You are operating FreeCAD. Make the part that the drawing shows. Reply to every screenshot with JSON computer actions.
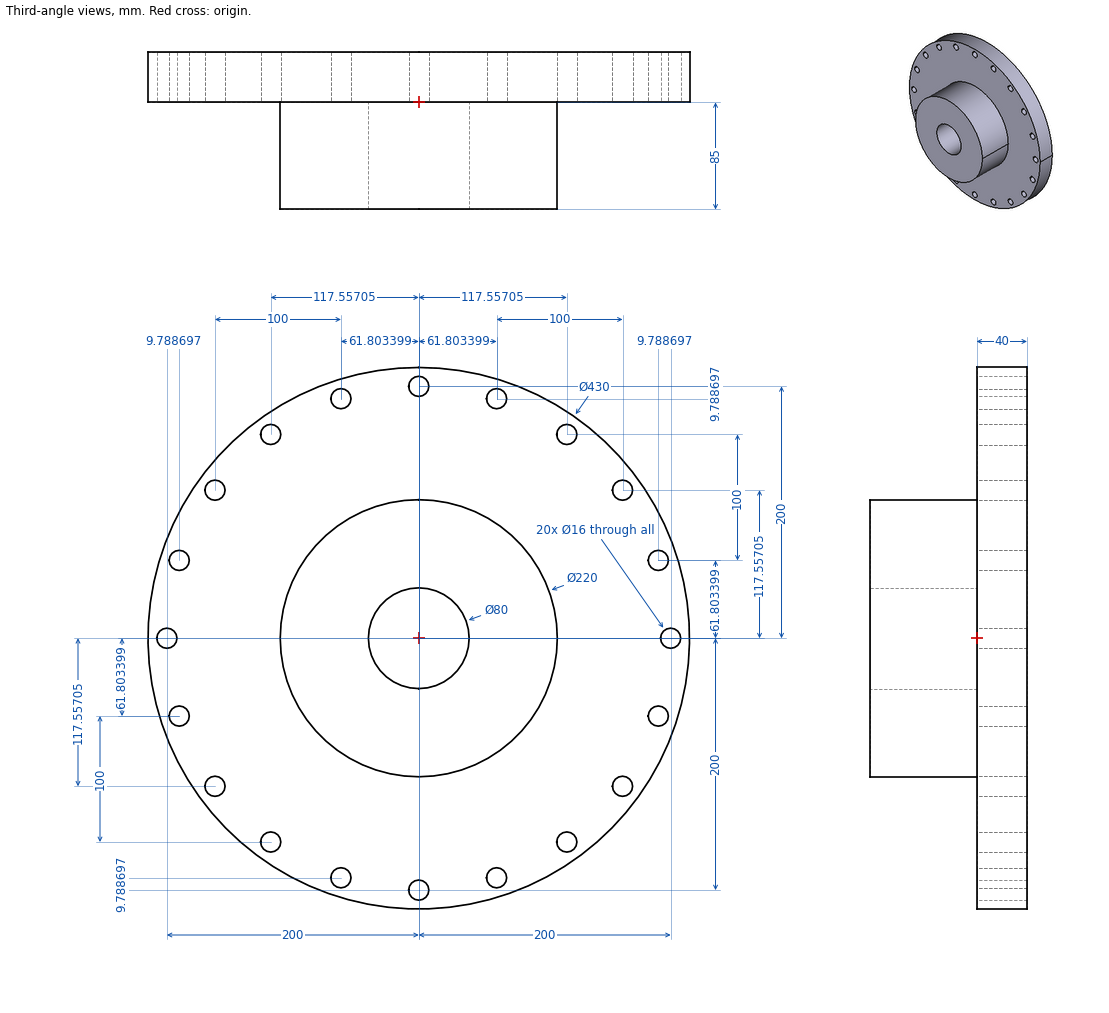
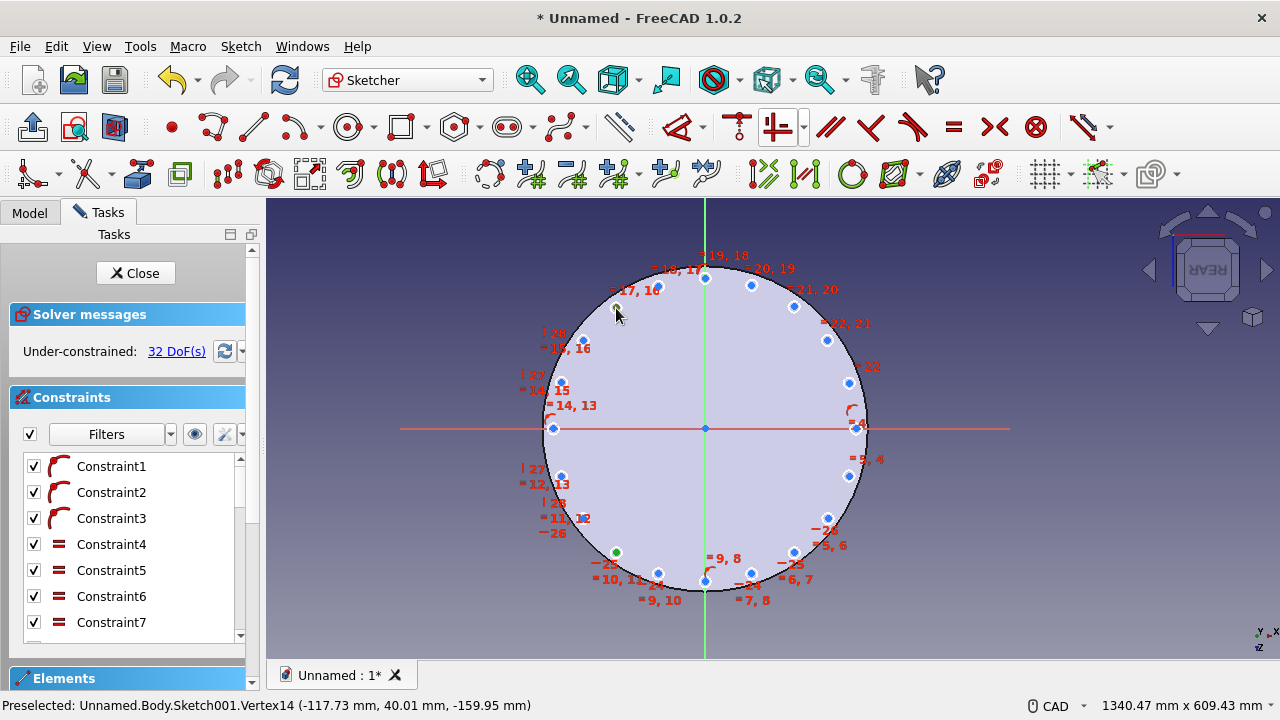
{"action": "key", "text": "v"}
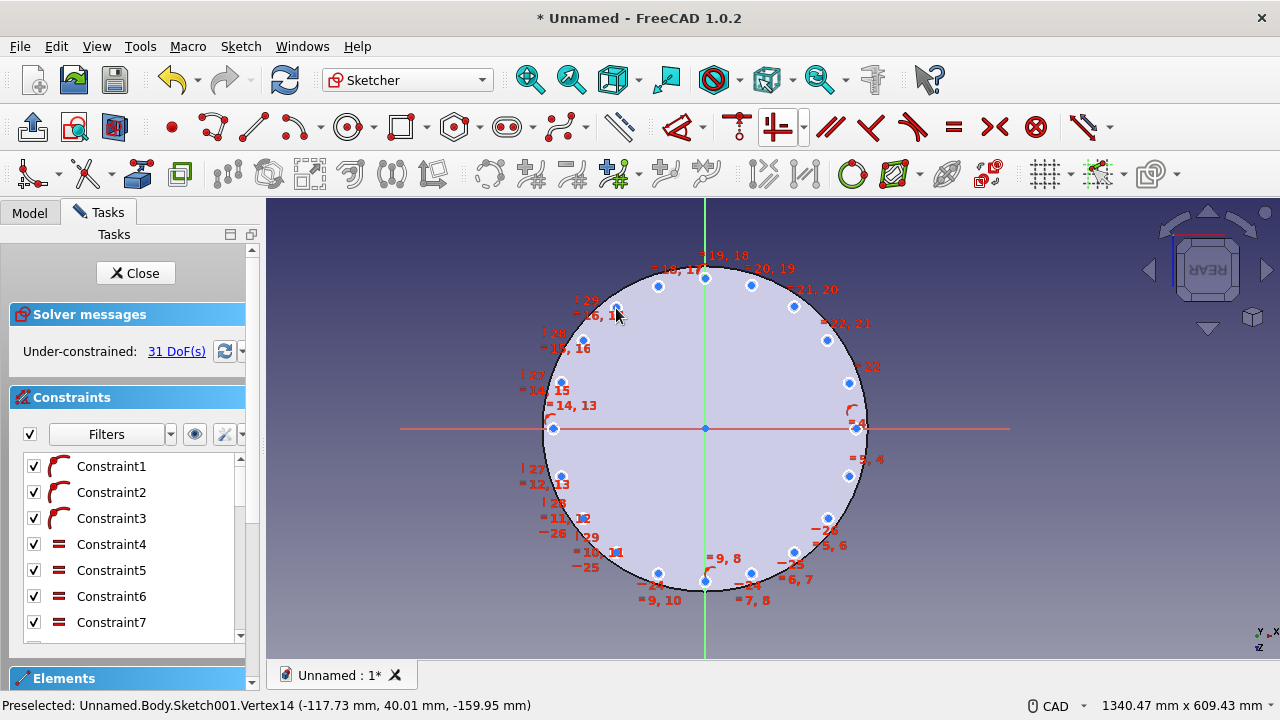
{"action": "left_click", "coordinate": [659, 286]}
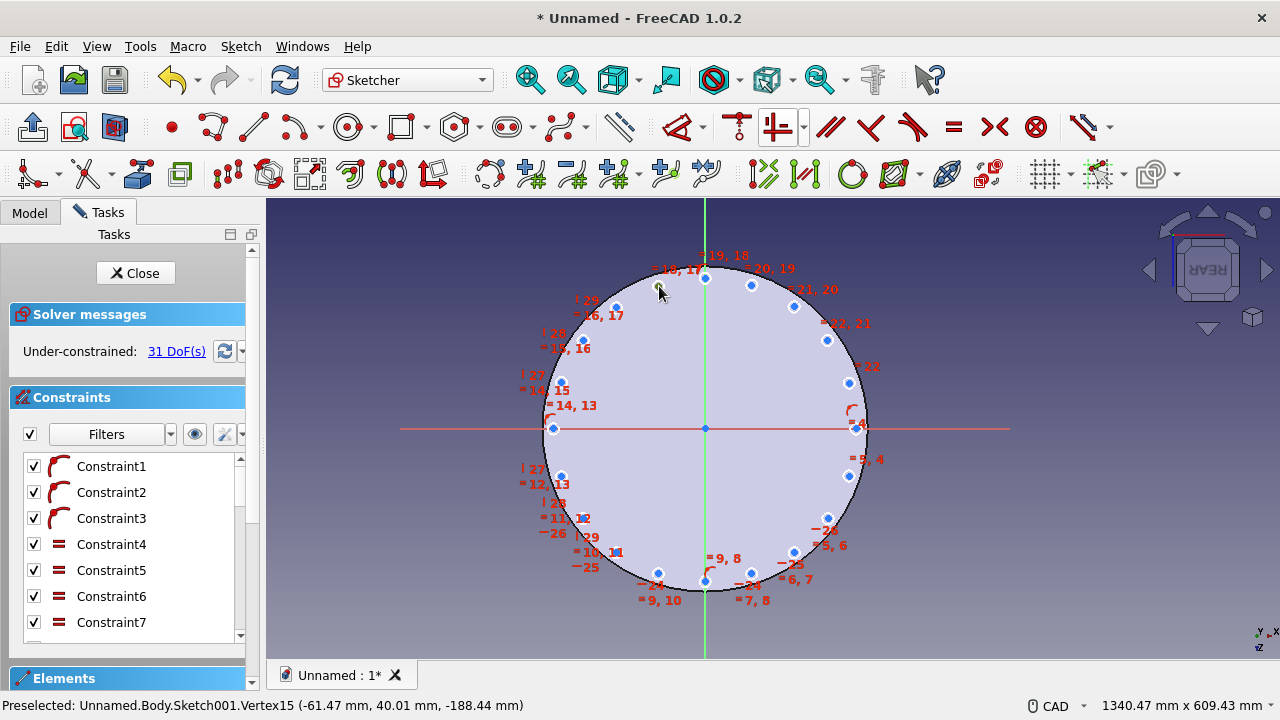
{"action": "left_click", "coordinate": [752, 285]}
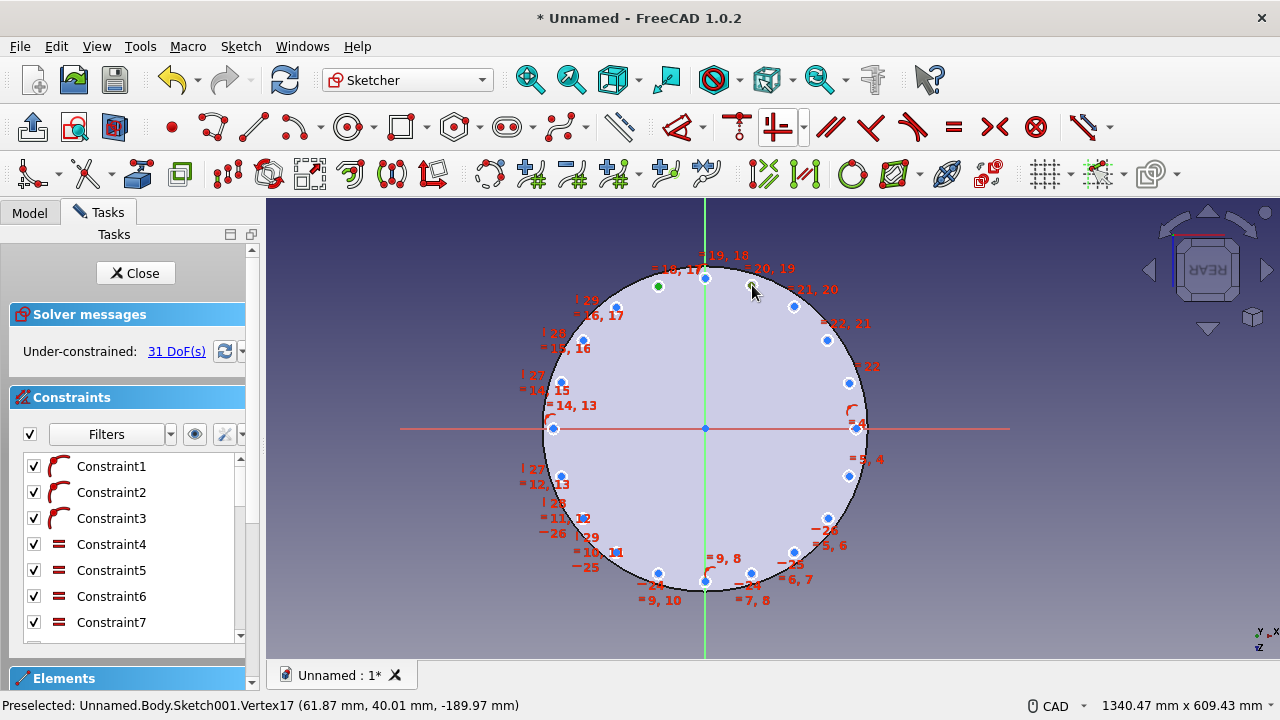
{"action": "key", "text": "h"}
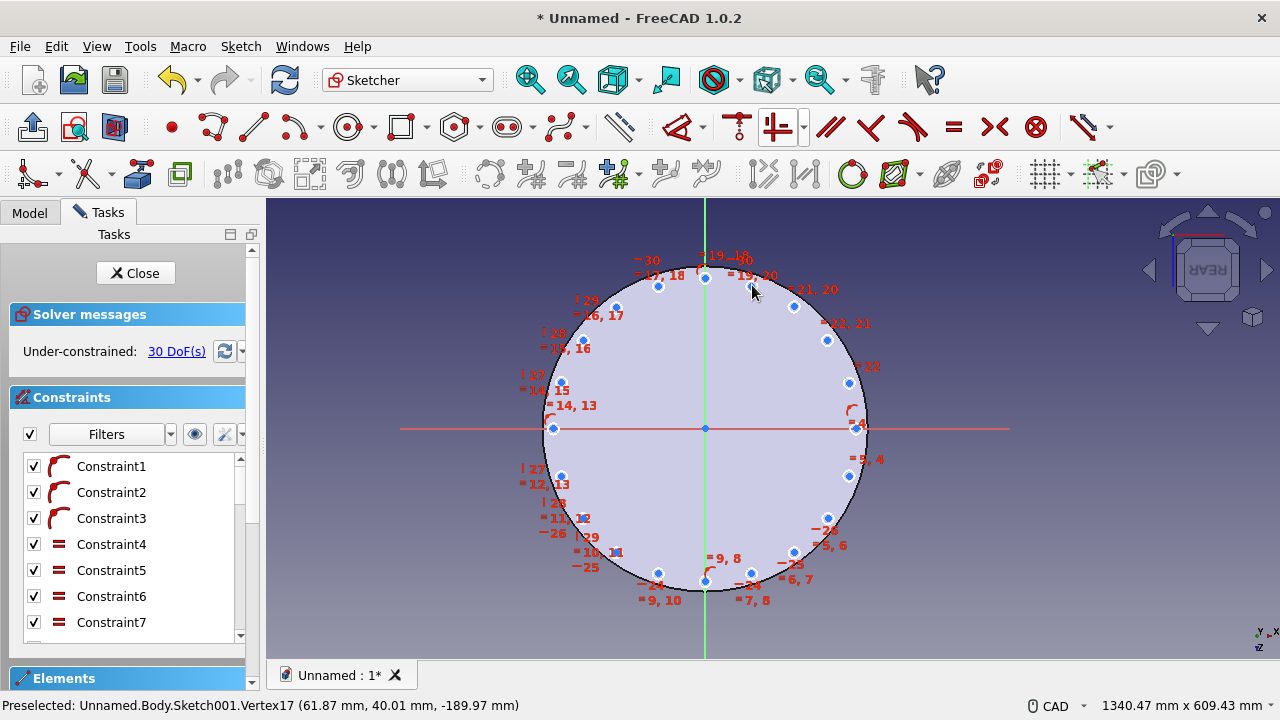
{"action": "scroll", "coordinate": [616, 308], "scroll_direction": "up", "scroll_amount": 4}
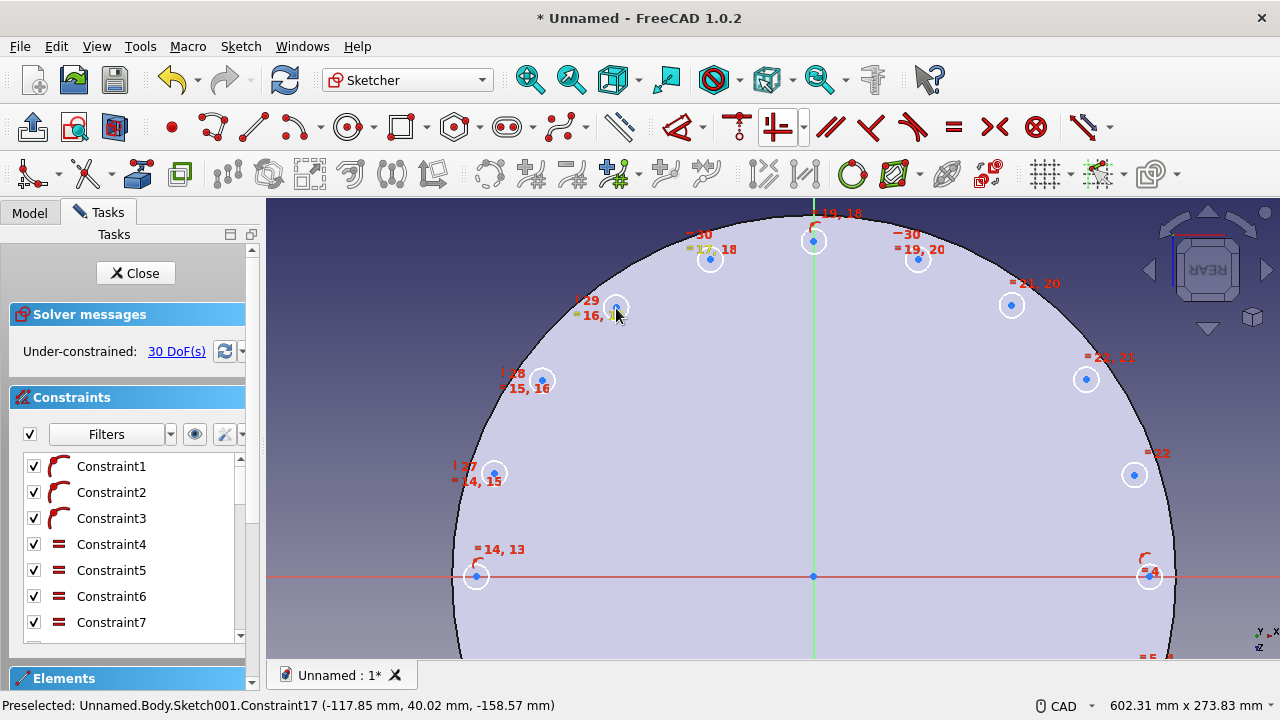
{"action": "scroll", "coordinate": [616, 308], "scroll_direction": "up", "scroll_amount": 4}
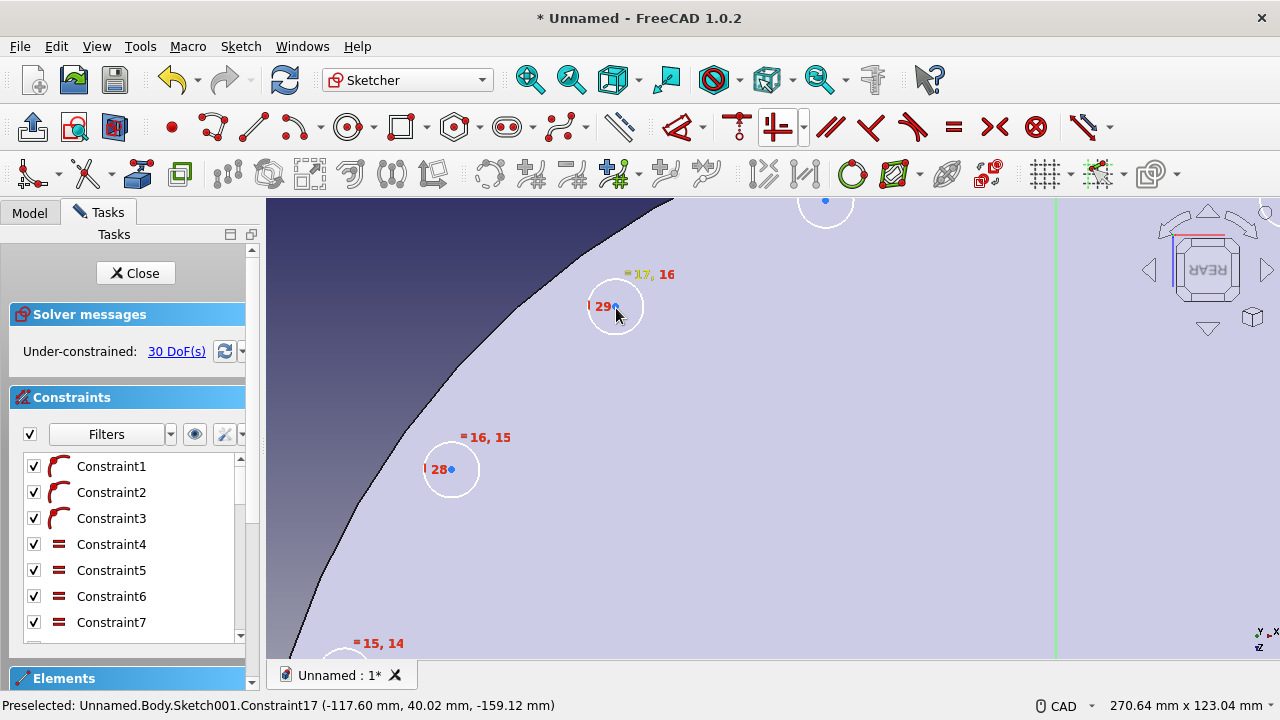
{"action": "left_click", "coordinate": [616, 307]}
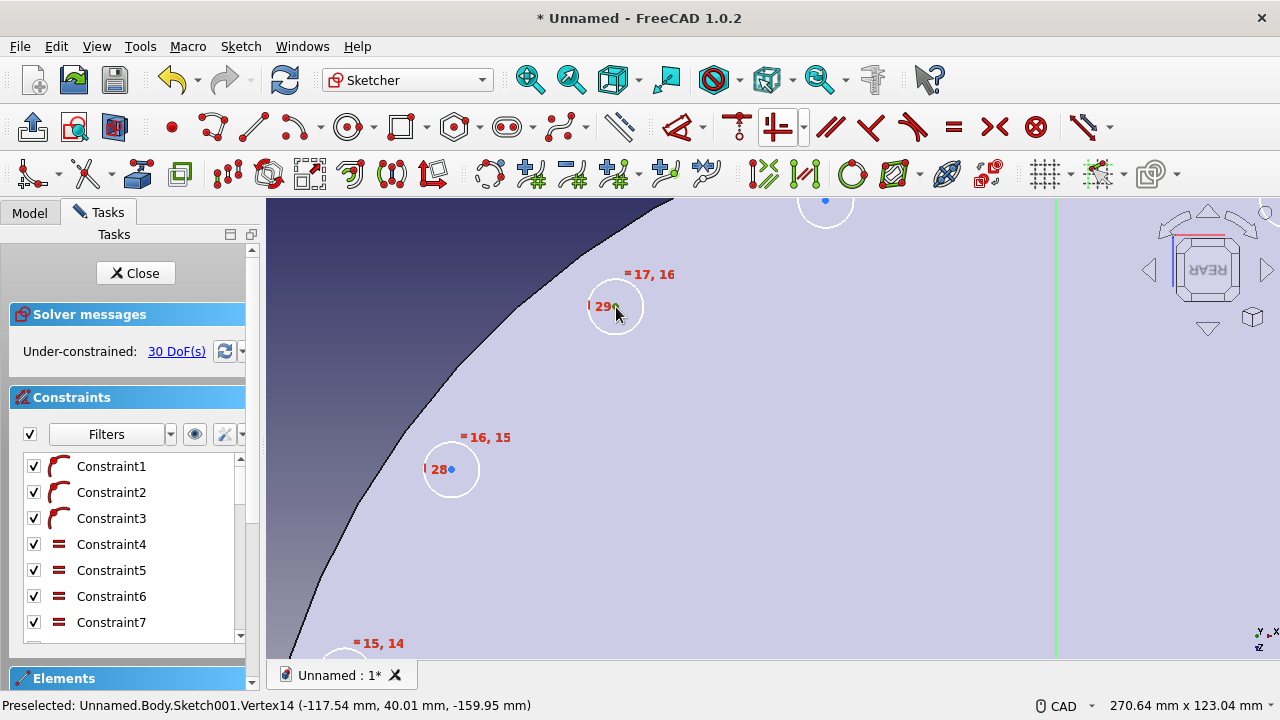
{"action": "scroll", "coordinate": [616, 308], "scroll_direction": "down", "scroll_amount": 8}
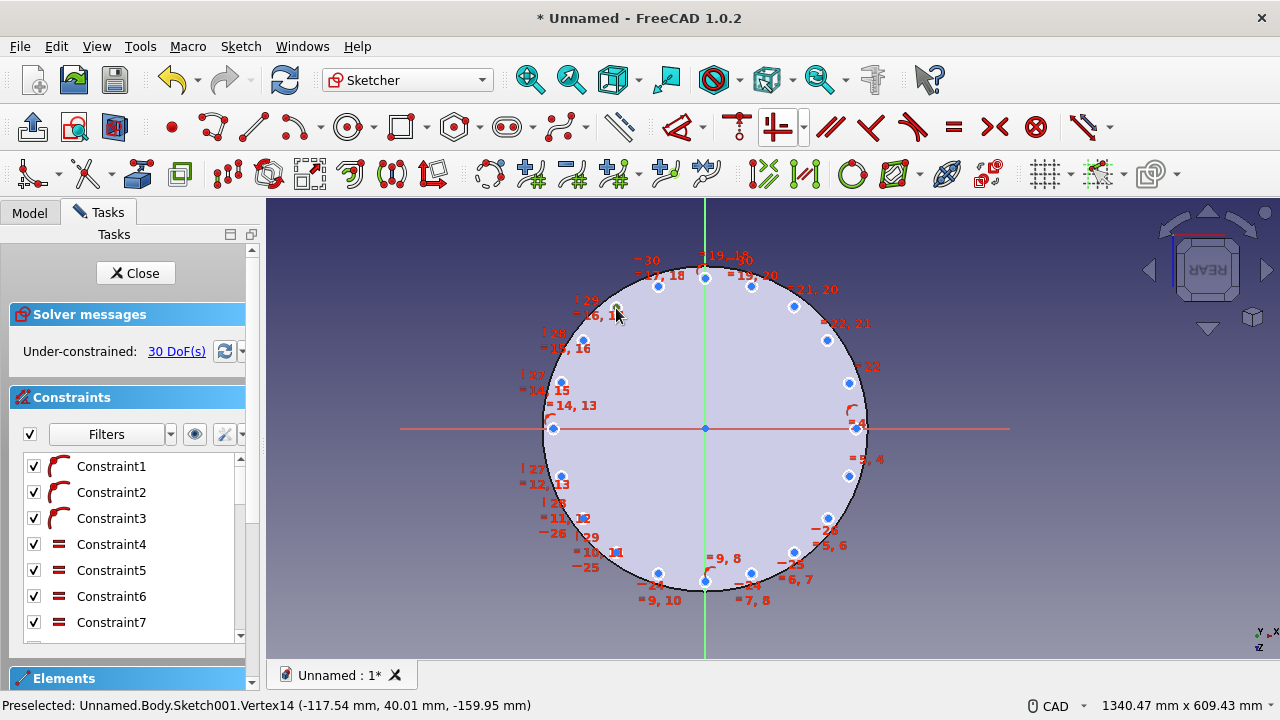
{"action": "left_click", "coordinate": [794, 307]}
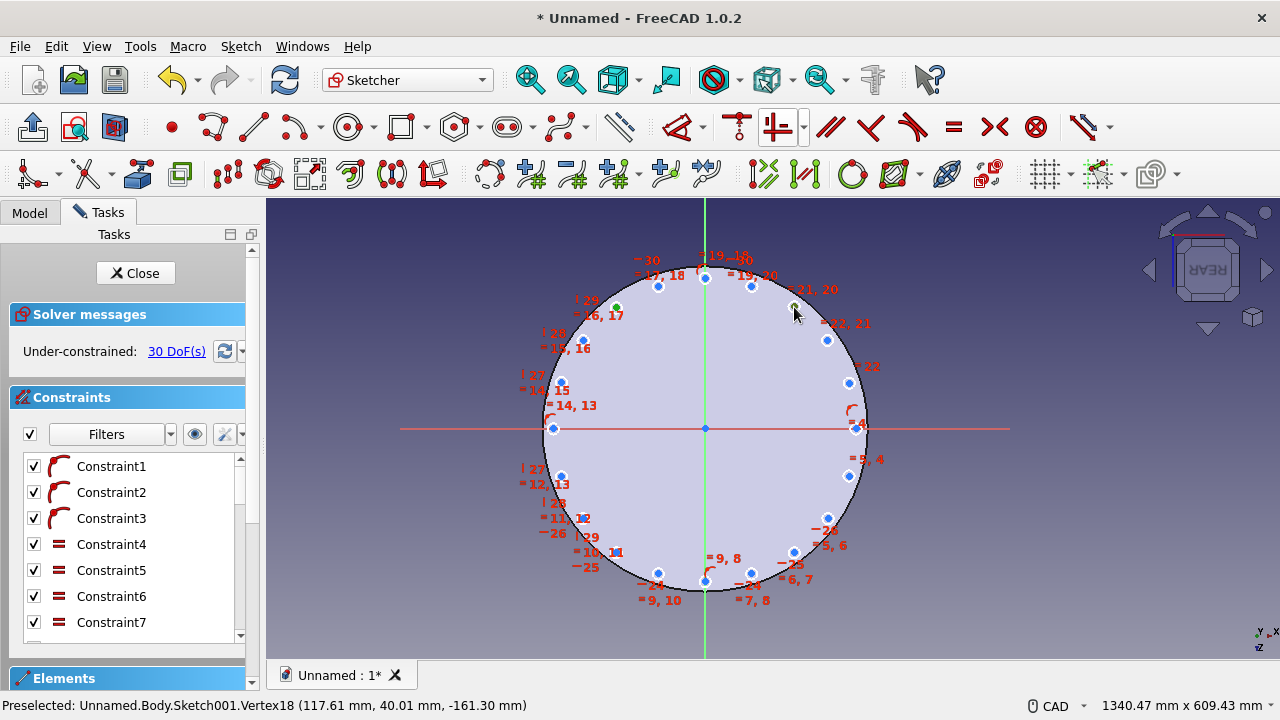
{"action": "left_click", "coordinate": [804, 128]}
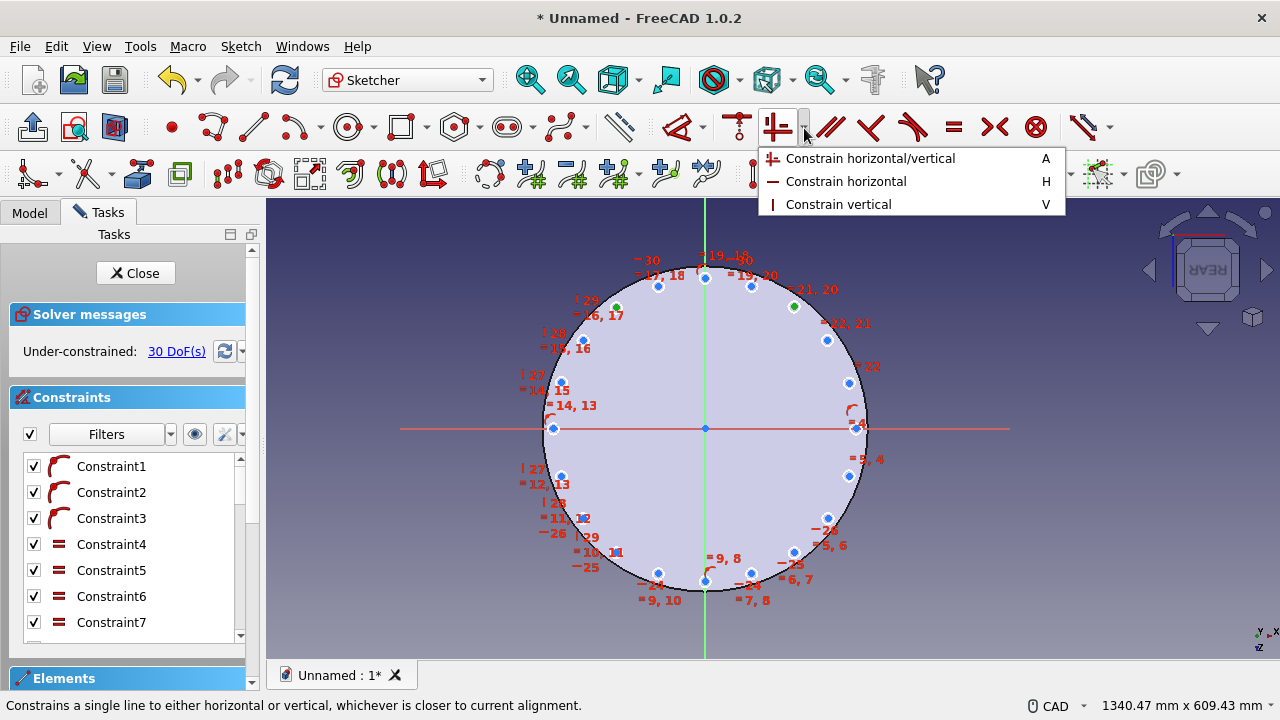
{"action": "left_click", "coordinate": [912, 182]}